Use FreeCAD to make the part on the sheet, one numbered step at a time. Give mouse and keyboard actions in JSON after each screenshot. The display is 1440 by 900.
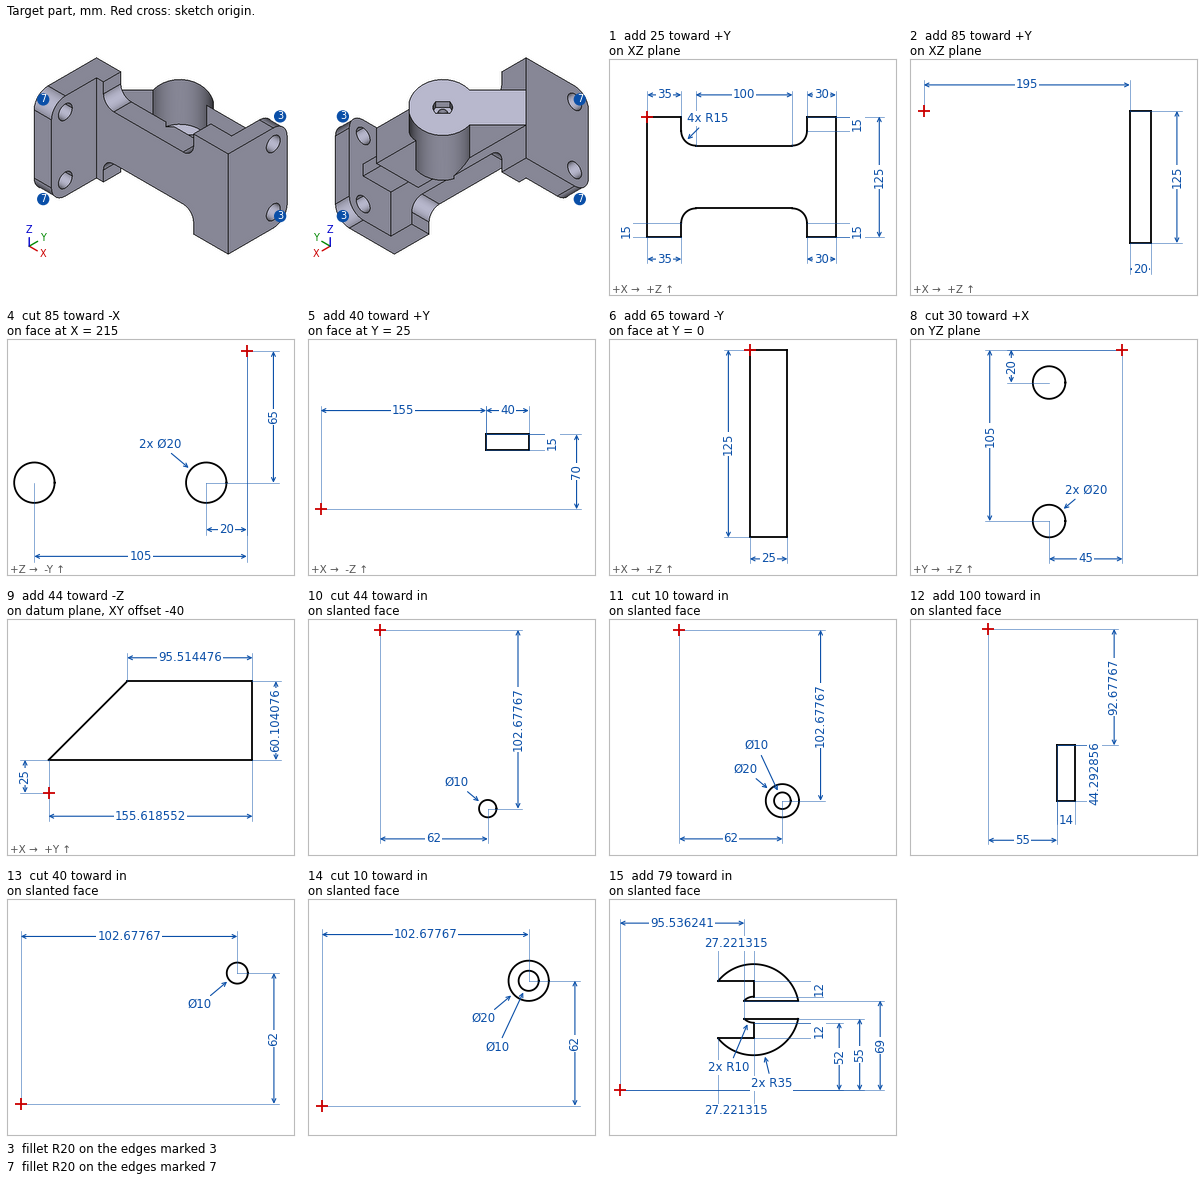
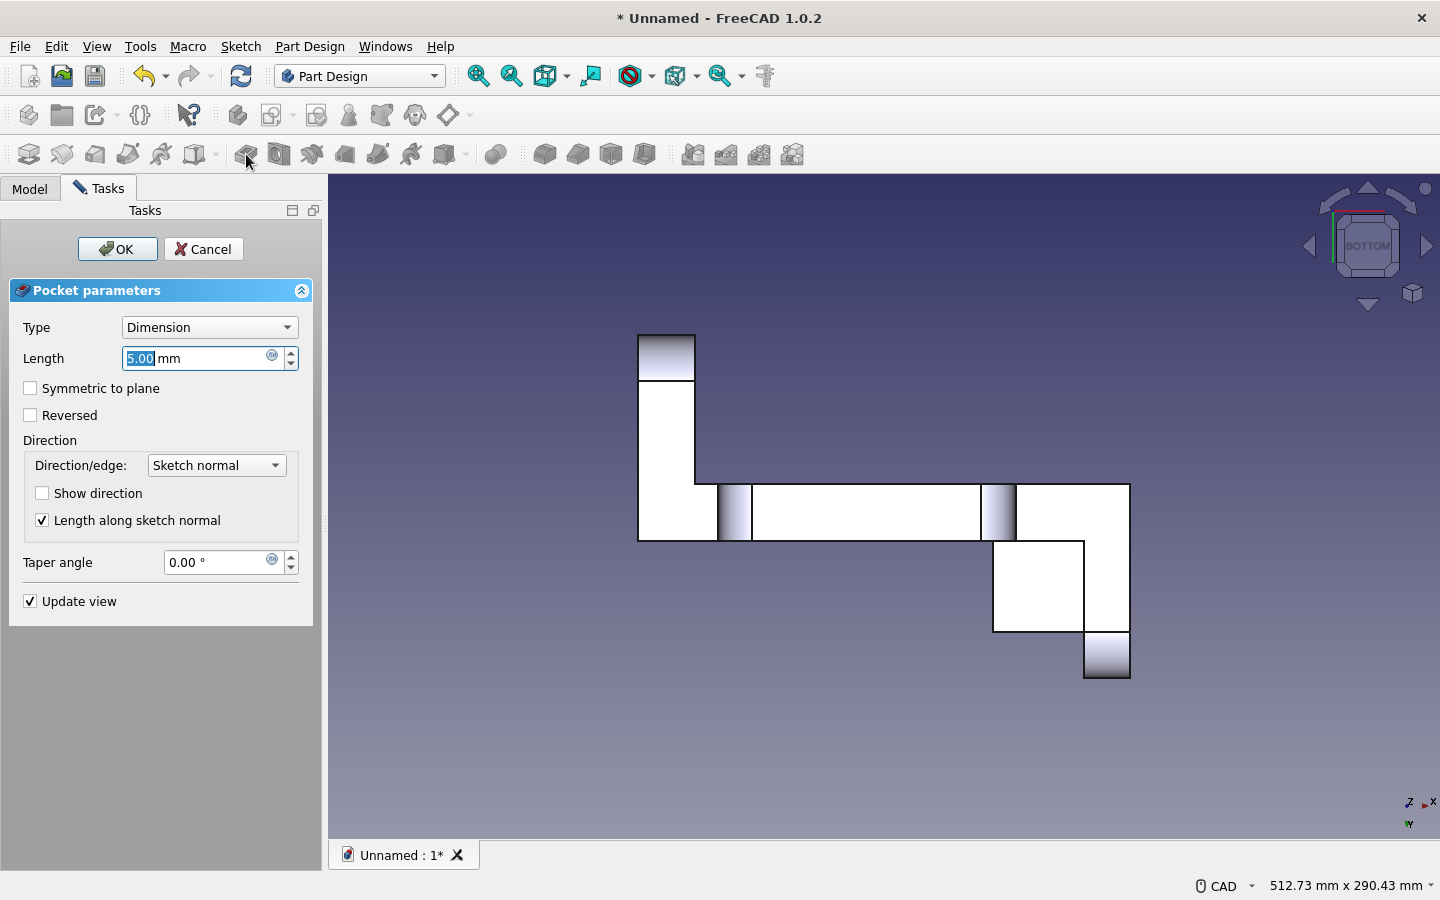
{"action": "type", "text": "30"}
{"action": "key", "text": "Tab"}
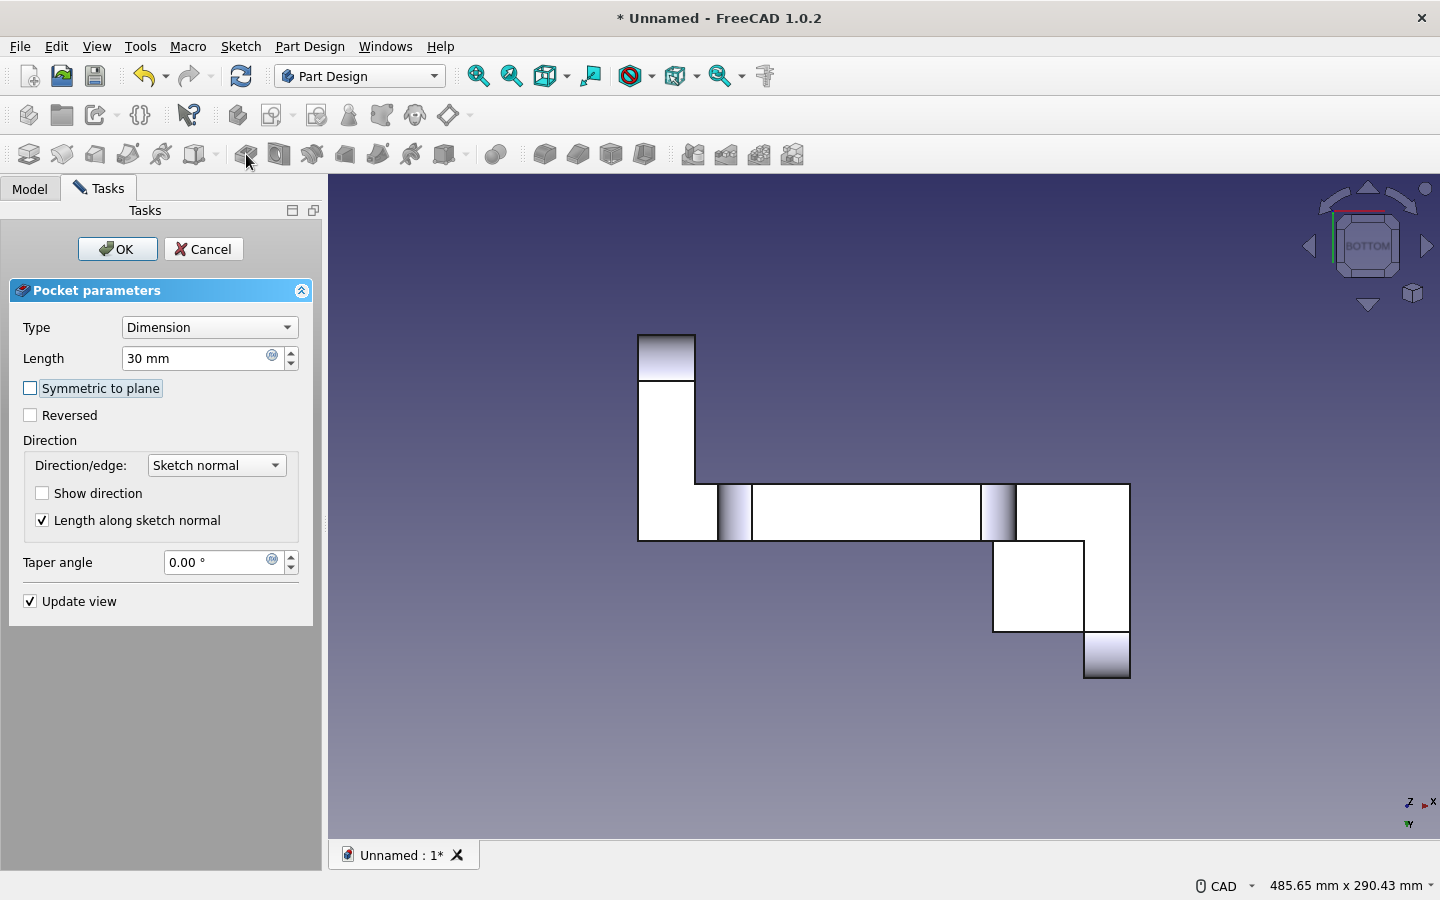
{"action": "left_click", "coordinate": [31, 415]}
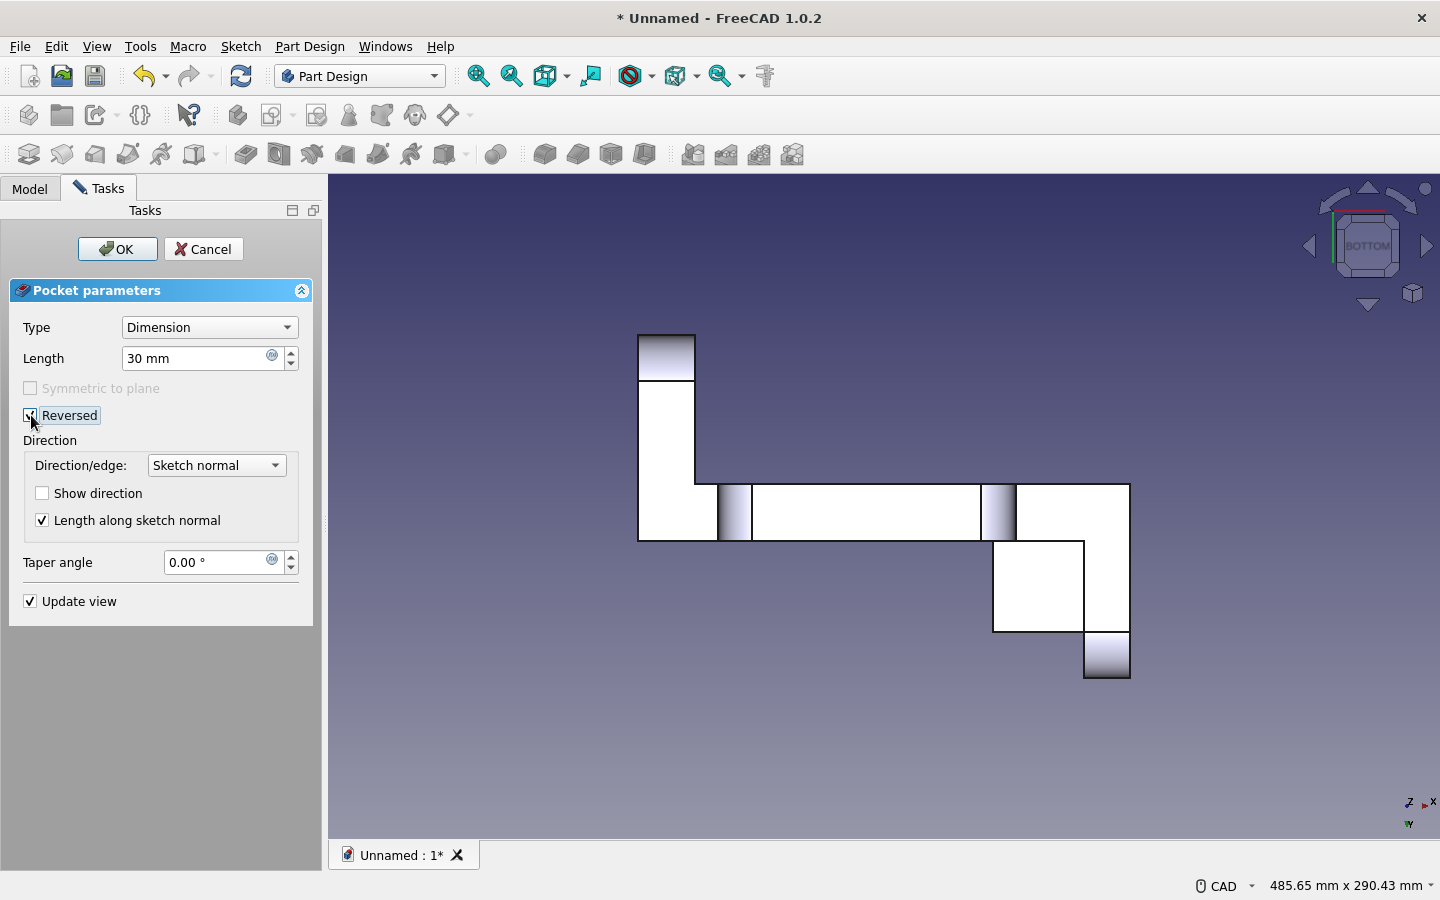
{"action": "left_click", "coordinate": [118, 249]}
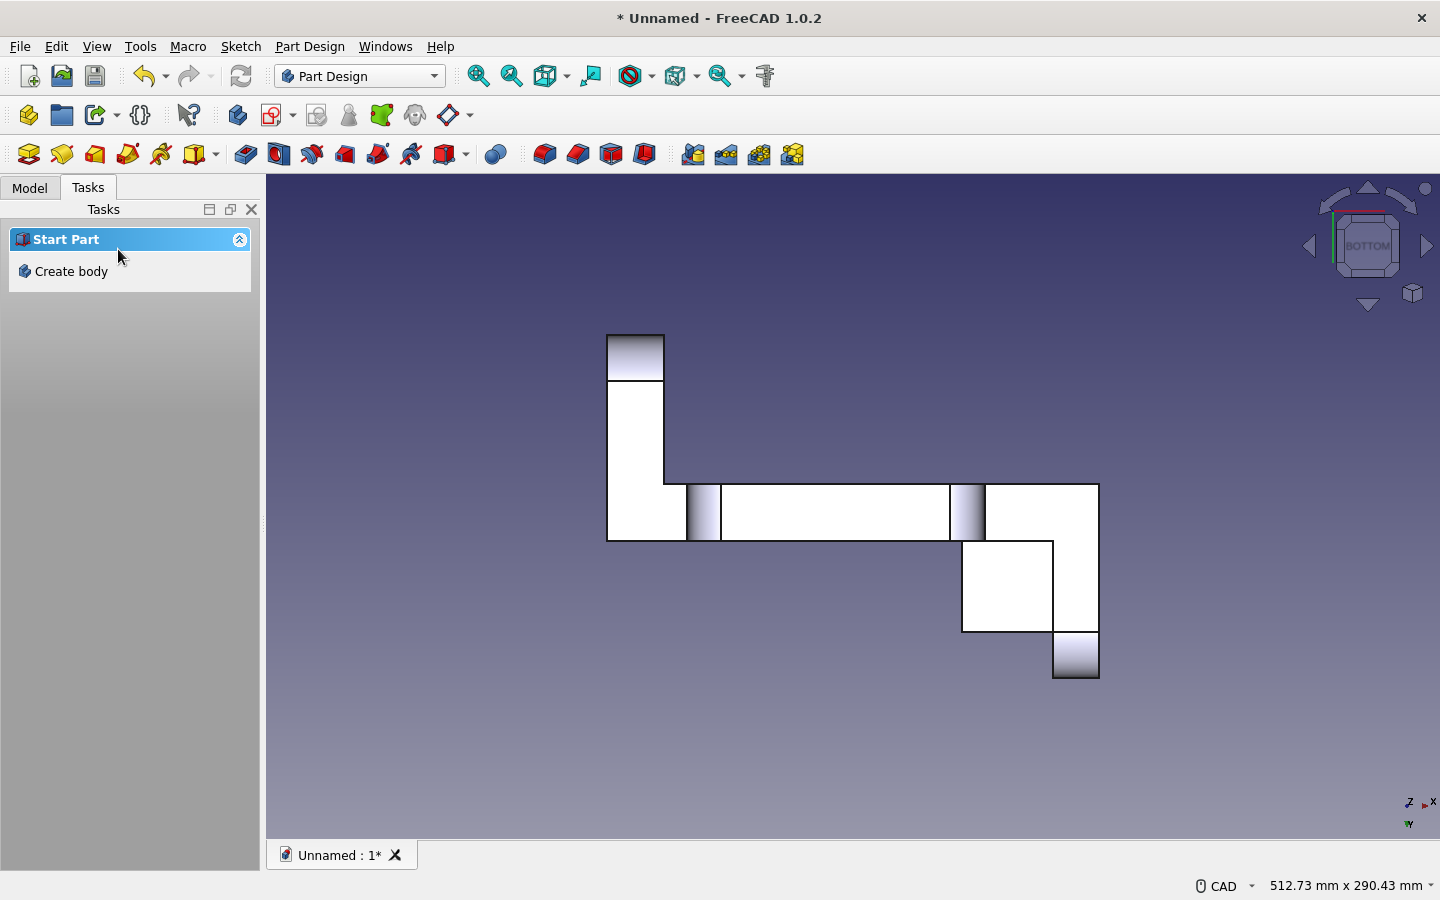
{"action": "left_click", "coordinate": [30, 188]}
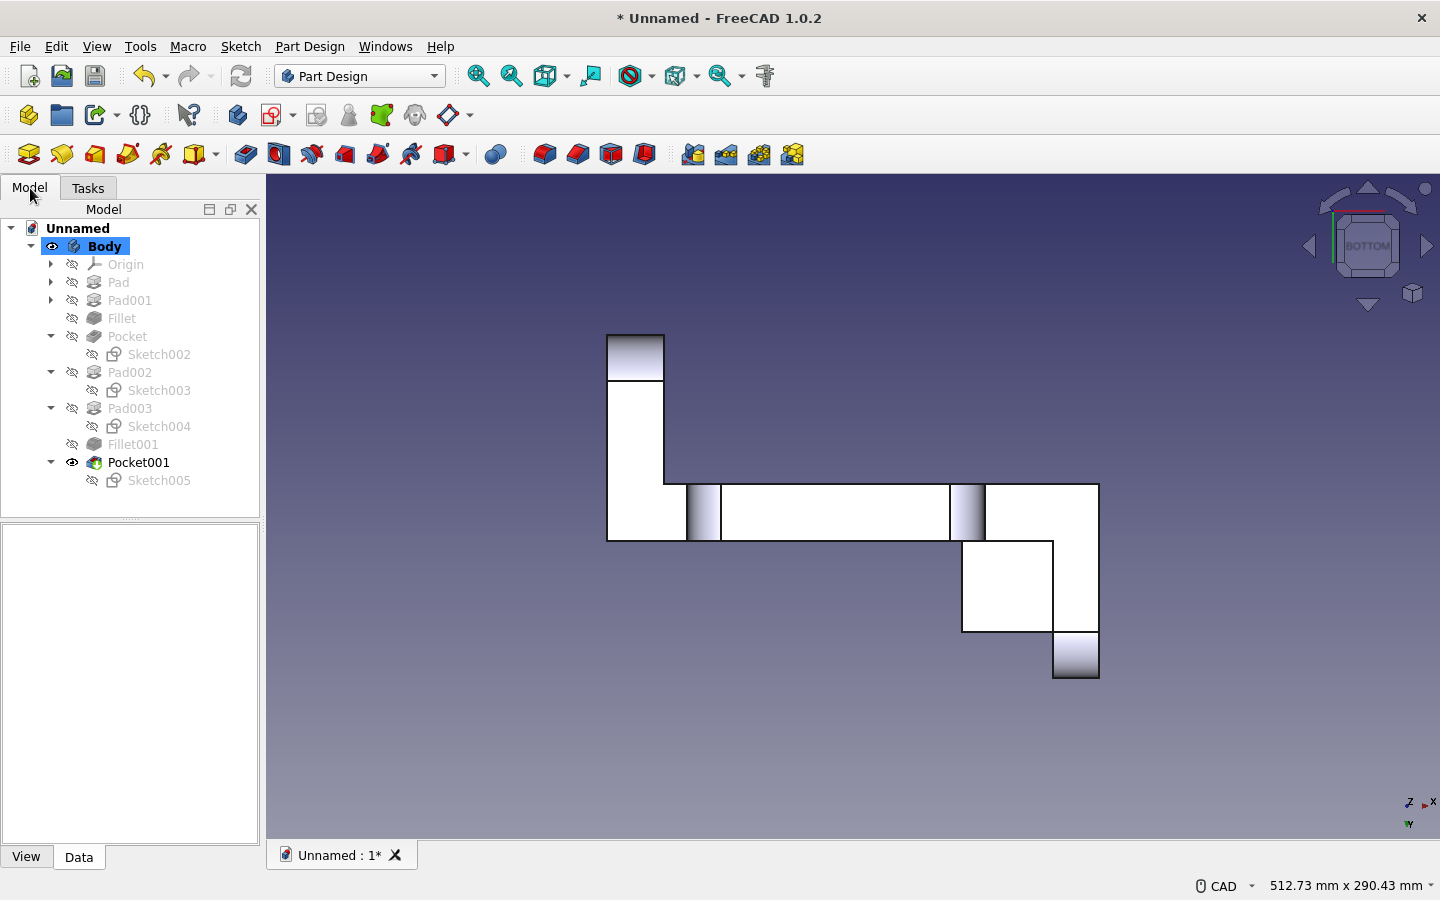
{"action": "left_click", "coordinate": [51, 264]}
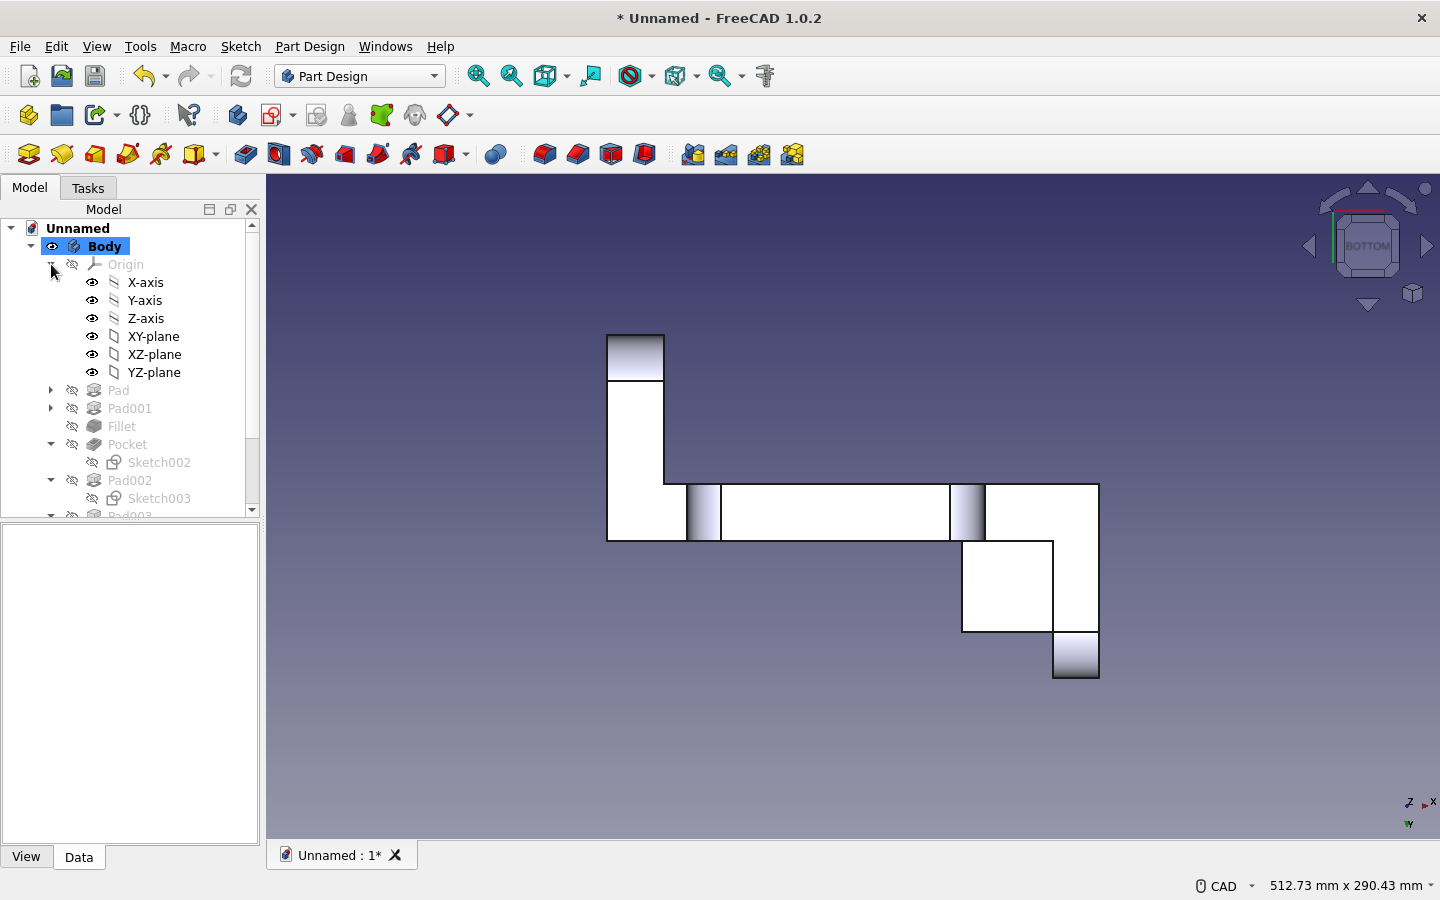
{"action": "left_click", "coordinate": [137, 336]}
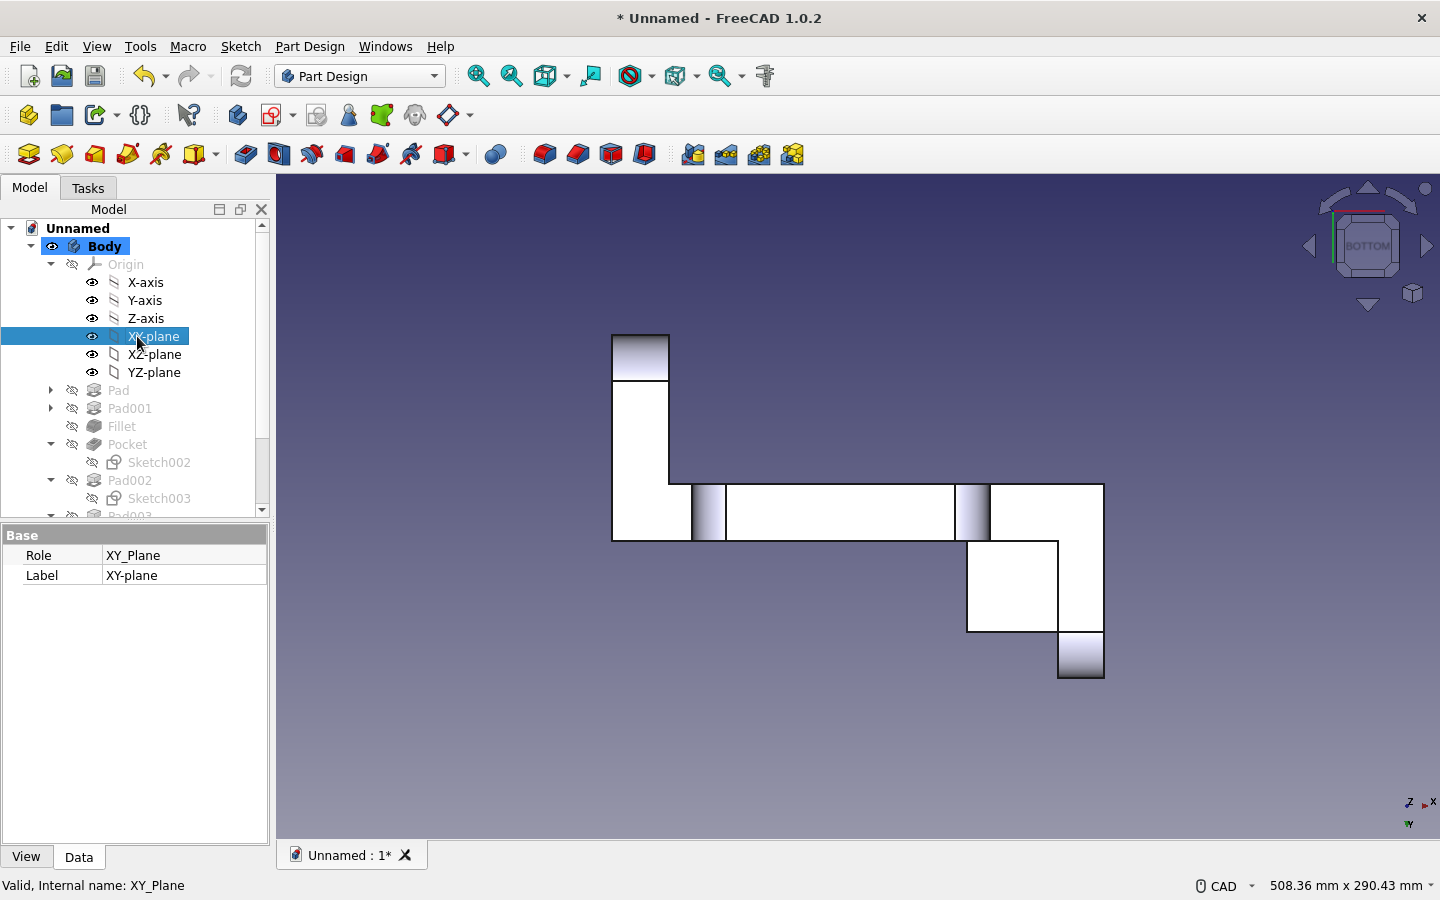
{"action": "left_click", "coordinate": [448, 116]}